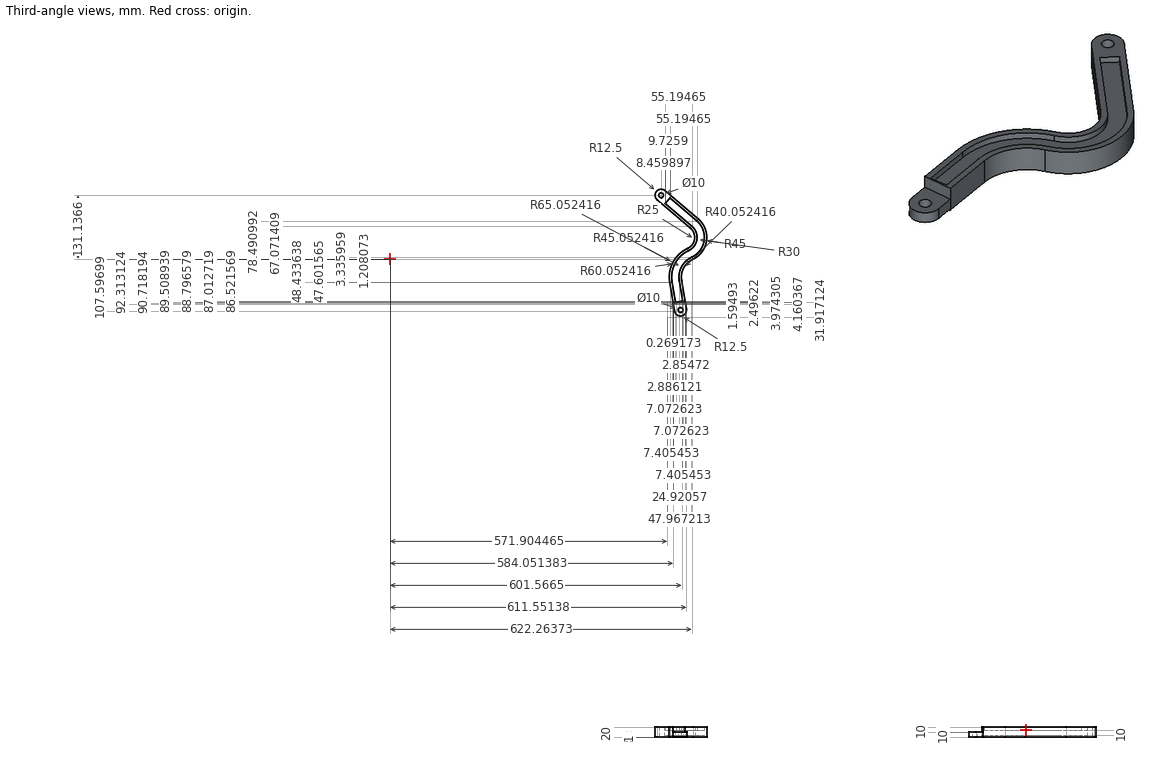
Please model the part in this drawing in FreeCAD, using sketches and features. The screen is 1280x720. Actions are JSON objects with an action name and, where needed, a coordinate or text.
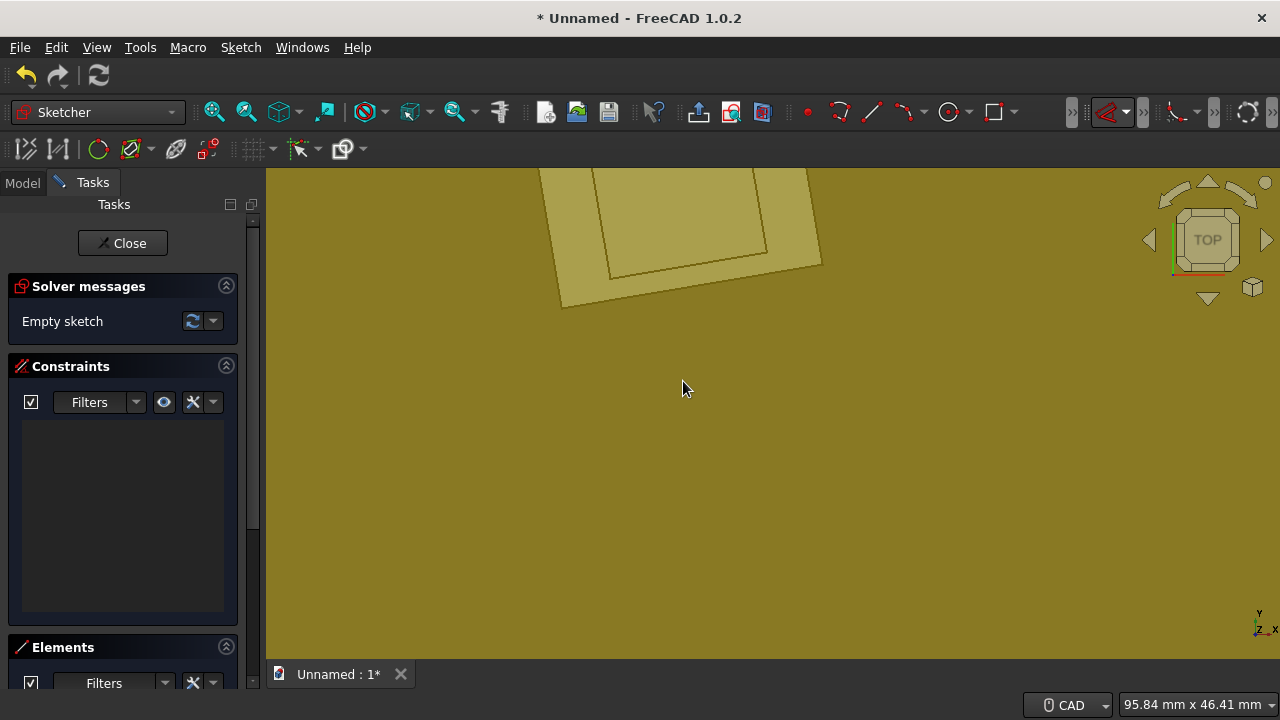
{"action": "key", "text": "g m"}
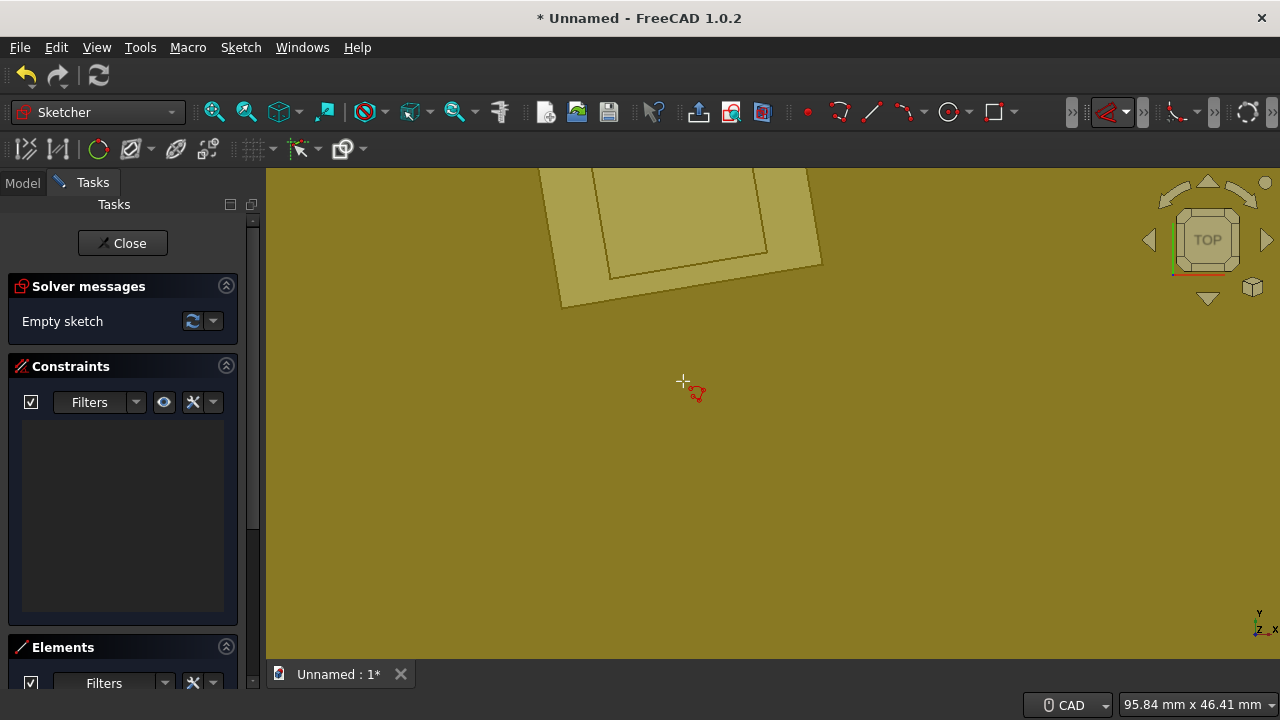
{"action": "left_click", "coordinate": [850, 426]}
{"action": "left_click", "coordinate": [820, 247]}
{"action": "left_click", "coordinate": [559, 289]}
{"action": "left_click", "coordinate": [589, 470]}
{"action": "right_click", "coordinate": [589, 470]}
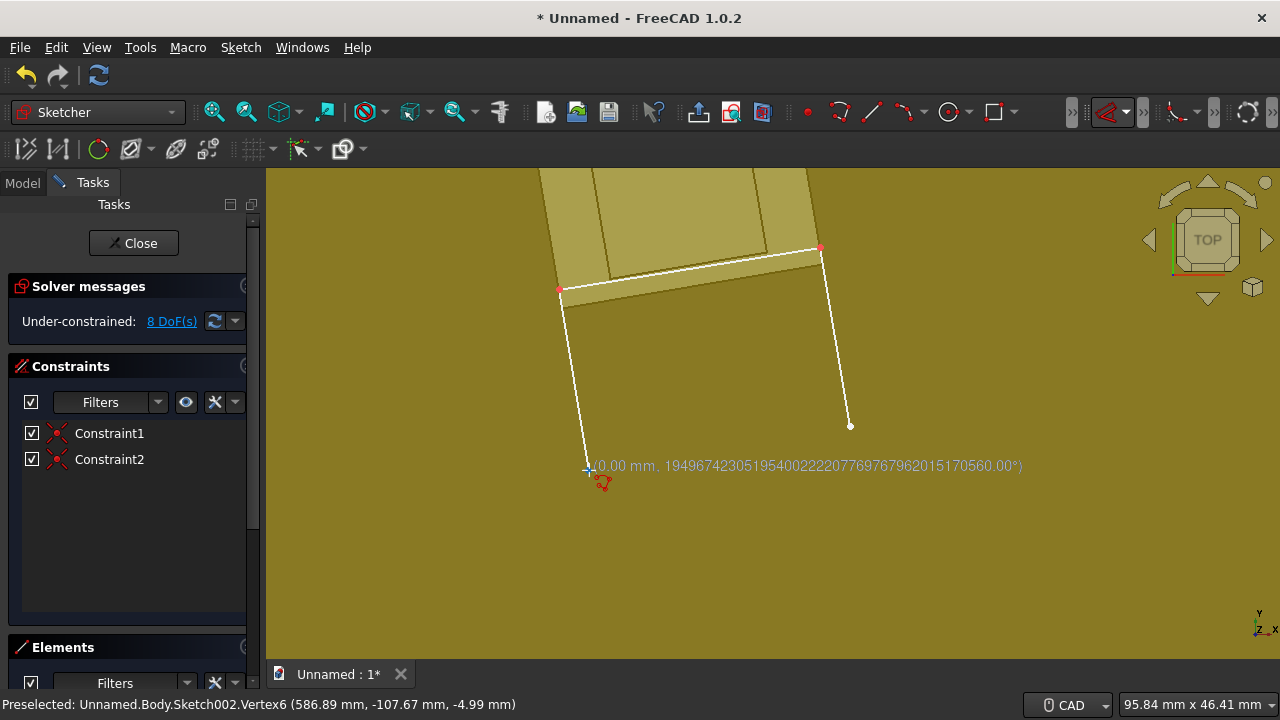
{"action": "left_click", "coordinate": [904, 112]}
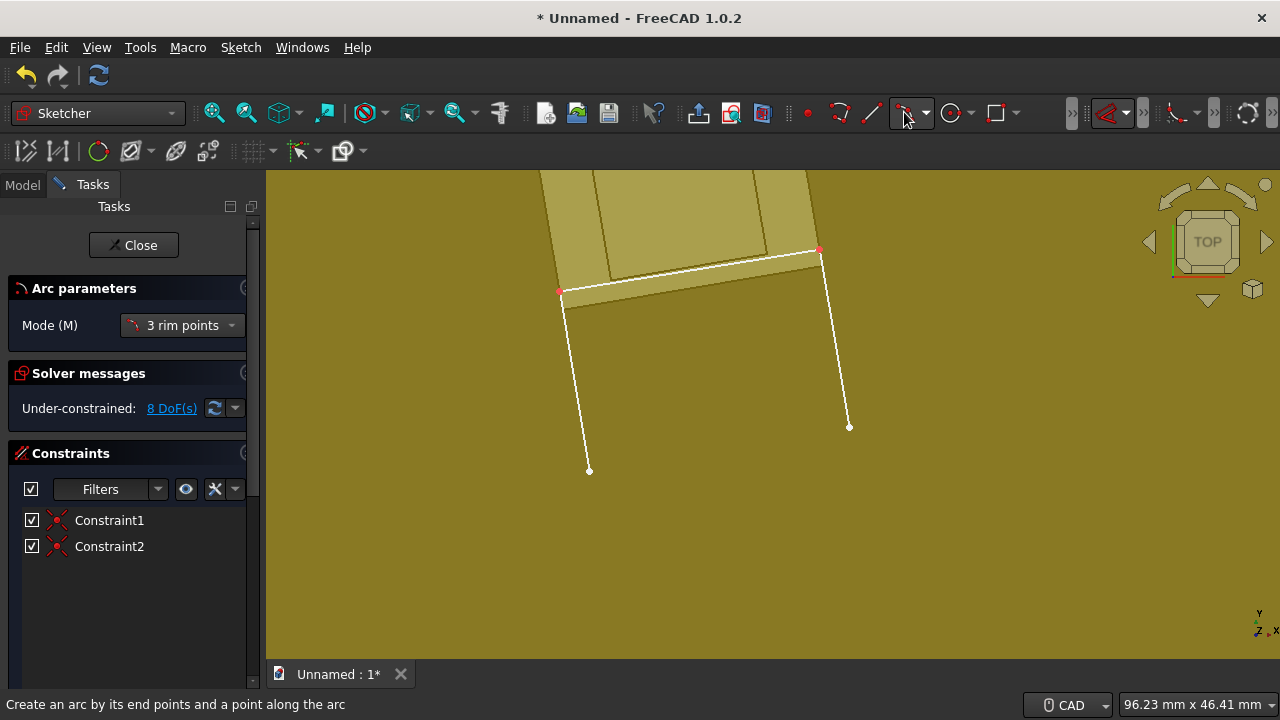
{"action": "left_click", "coordinate": [590, 472]}
{"action": "left_click", "coordinate": [850, 428]}
{"action": "left_click", "coordinate": [742, 579]}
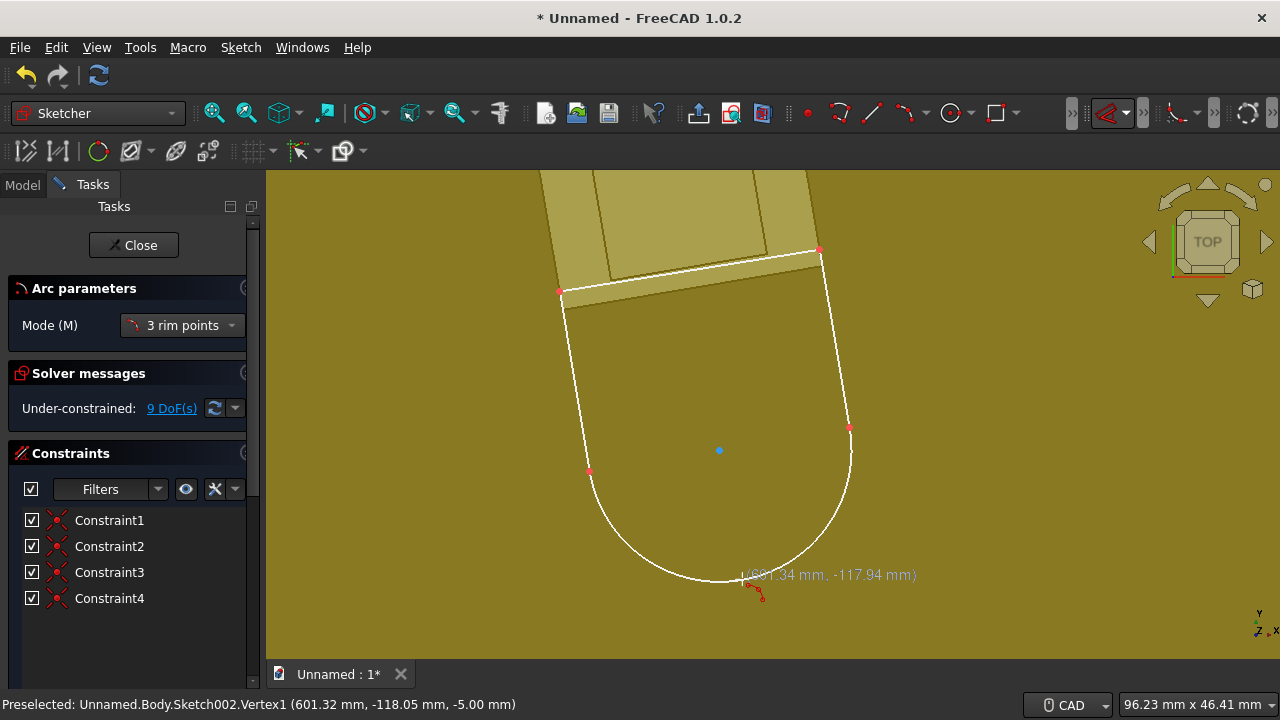
{"action": "key", "text": "g c"}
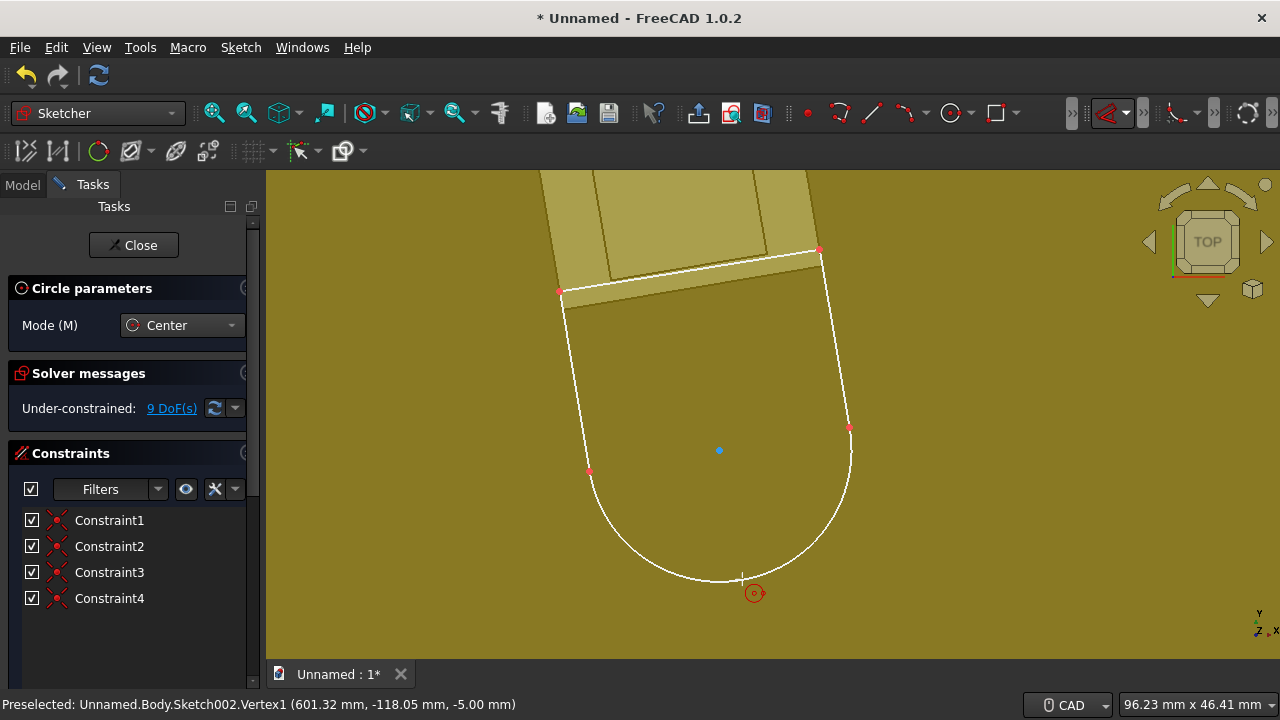
{"action": "left_click", "coordinate": [720, 449]}
{"action": "left_click", "coordinate": [757, 412]}
{"action": "key", "text": "Escape"}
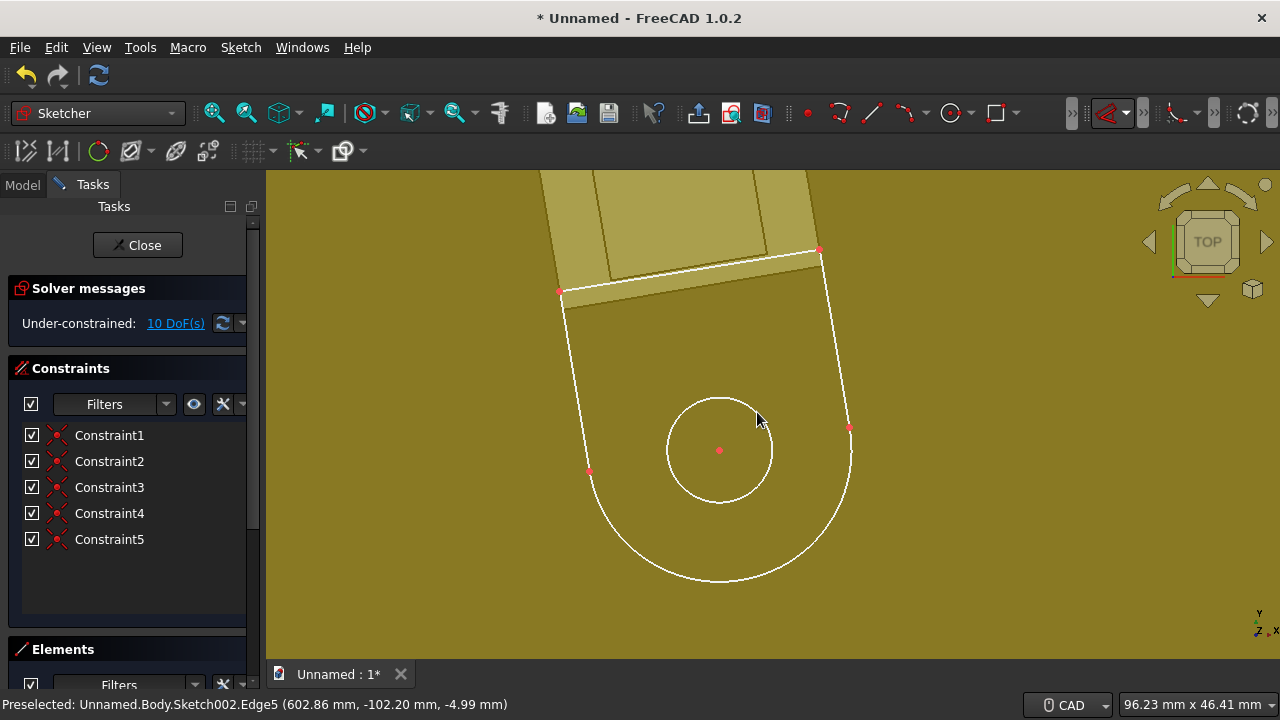
{"action": "left_click", "coordinate": [841, 374]}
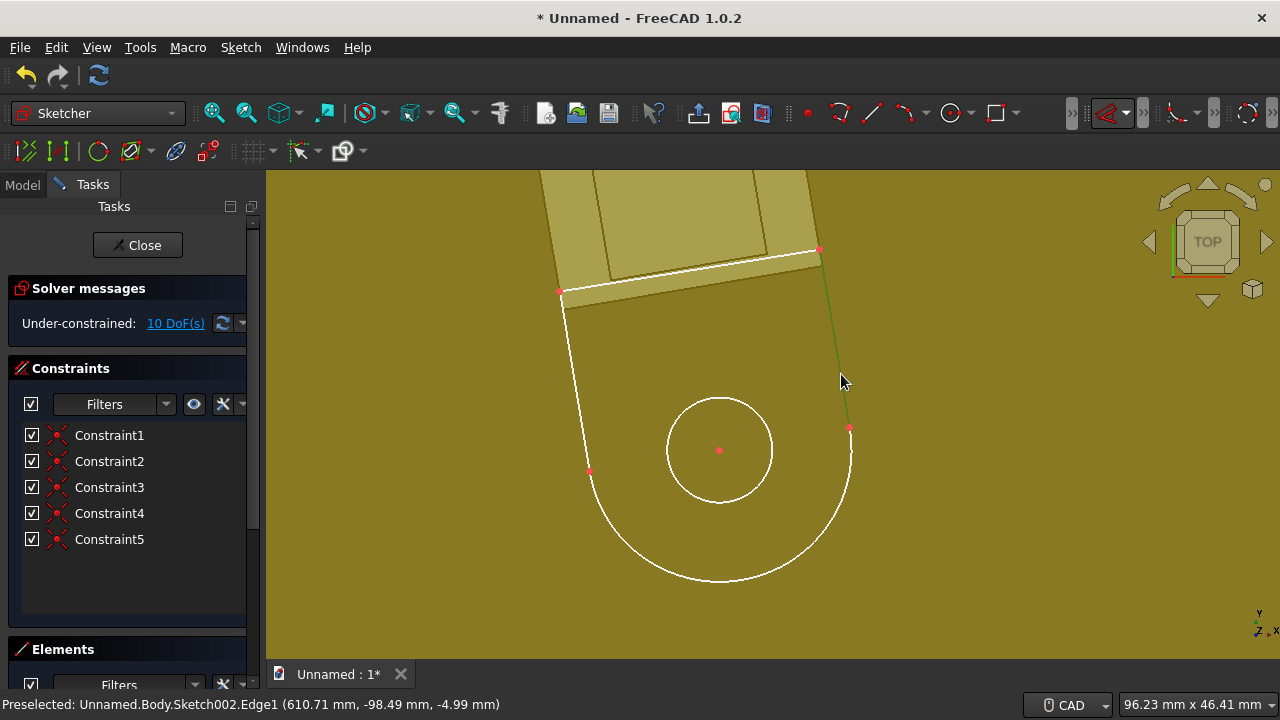
{"action": "left_click", "coordinate": [661, 568]}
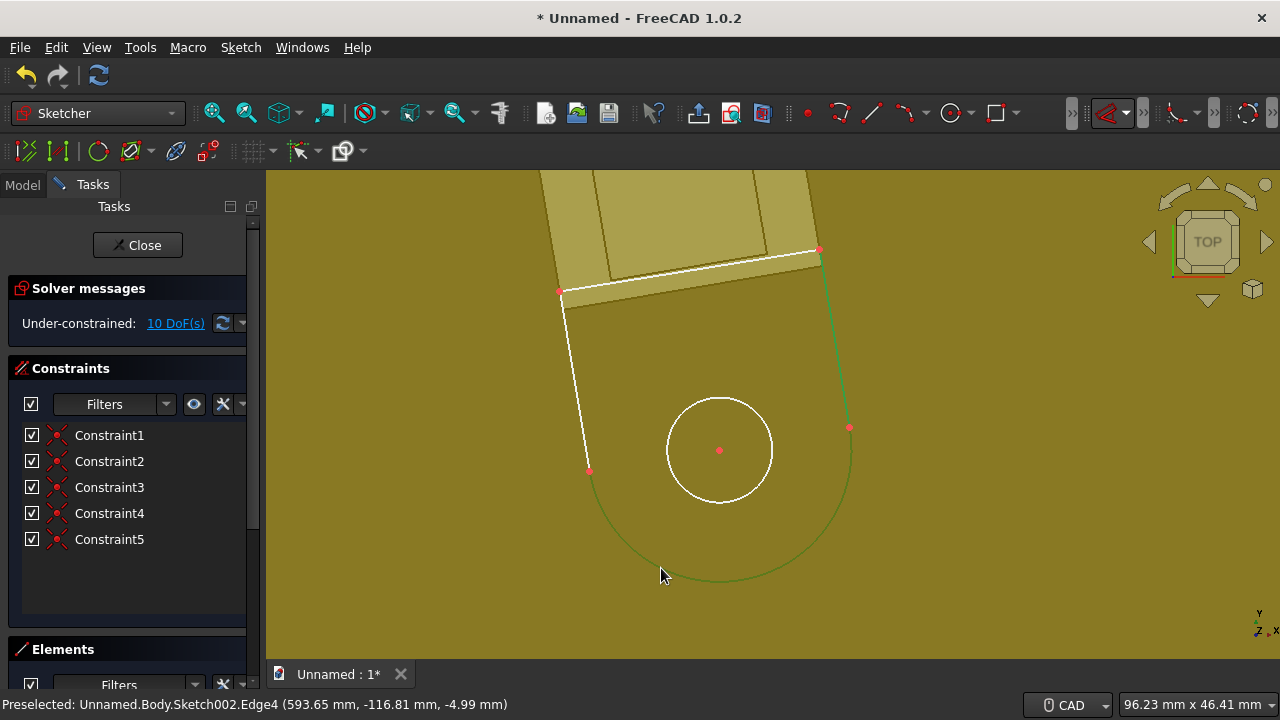
{"action": "key", "text": "t"}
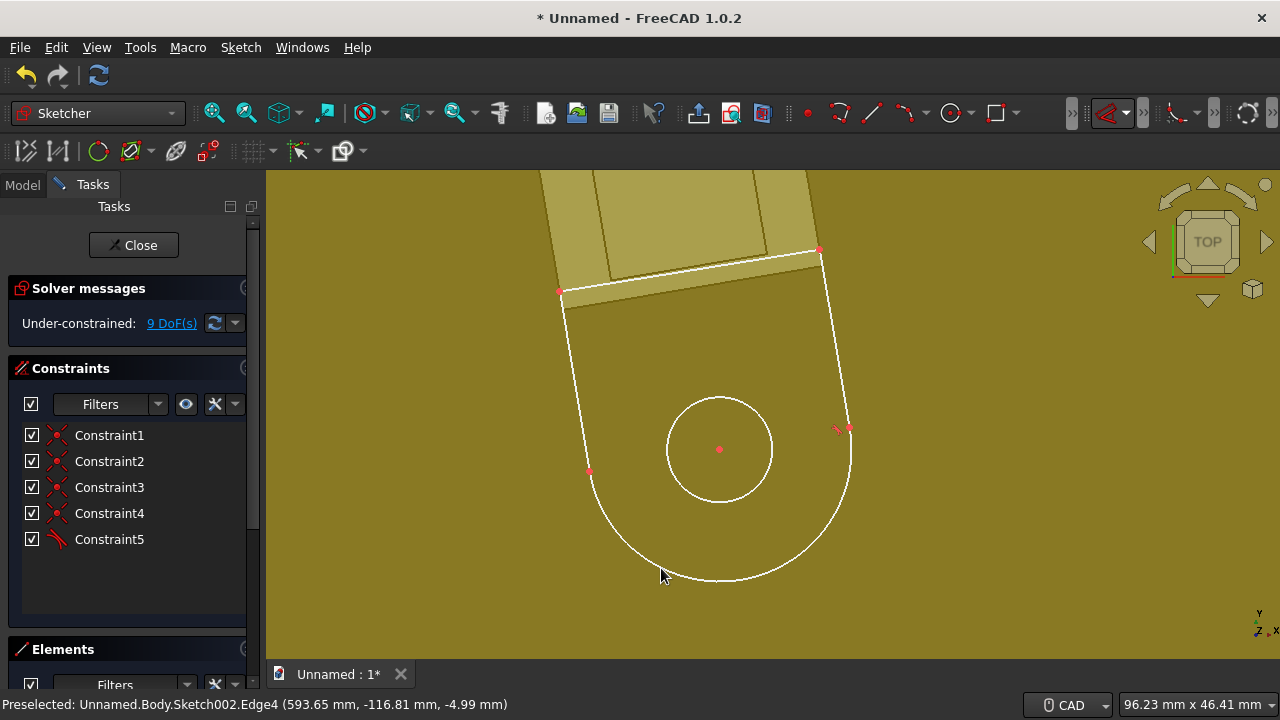
{"action": "left_click", "coordinate": [569, 346]}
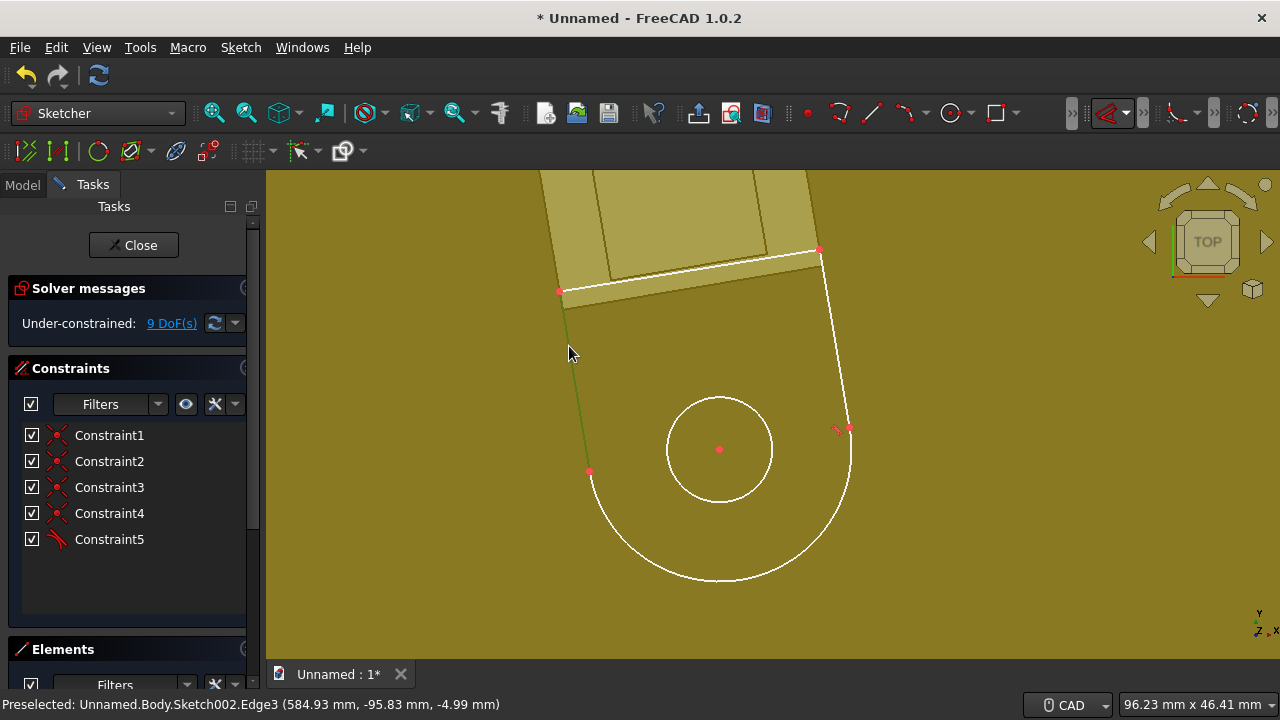
{"action": "left_click", "coordinate": [661, 568]}